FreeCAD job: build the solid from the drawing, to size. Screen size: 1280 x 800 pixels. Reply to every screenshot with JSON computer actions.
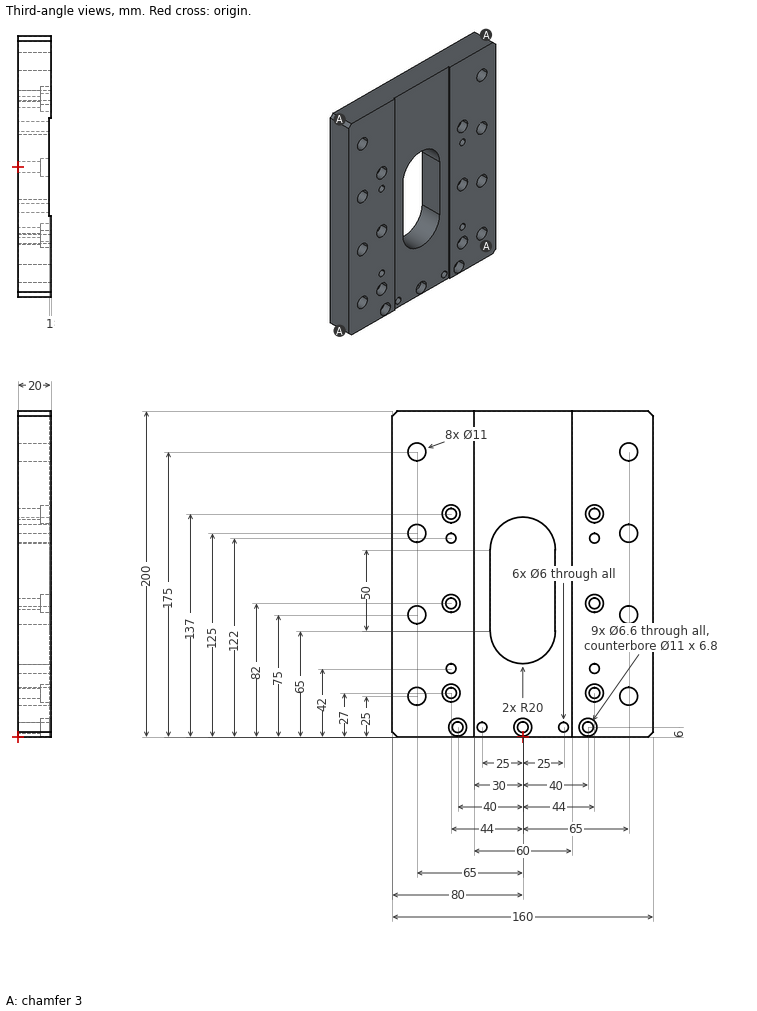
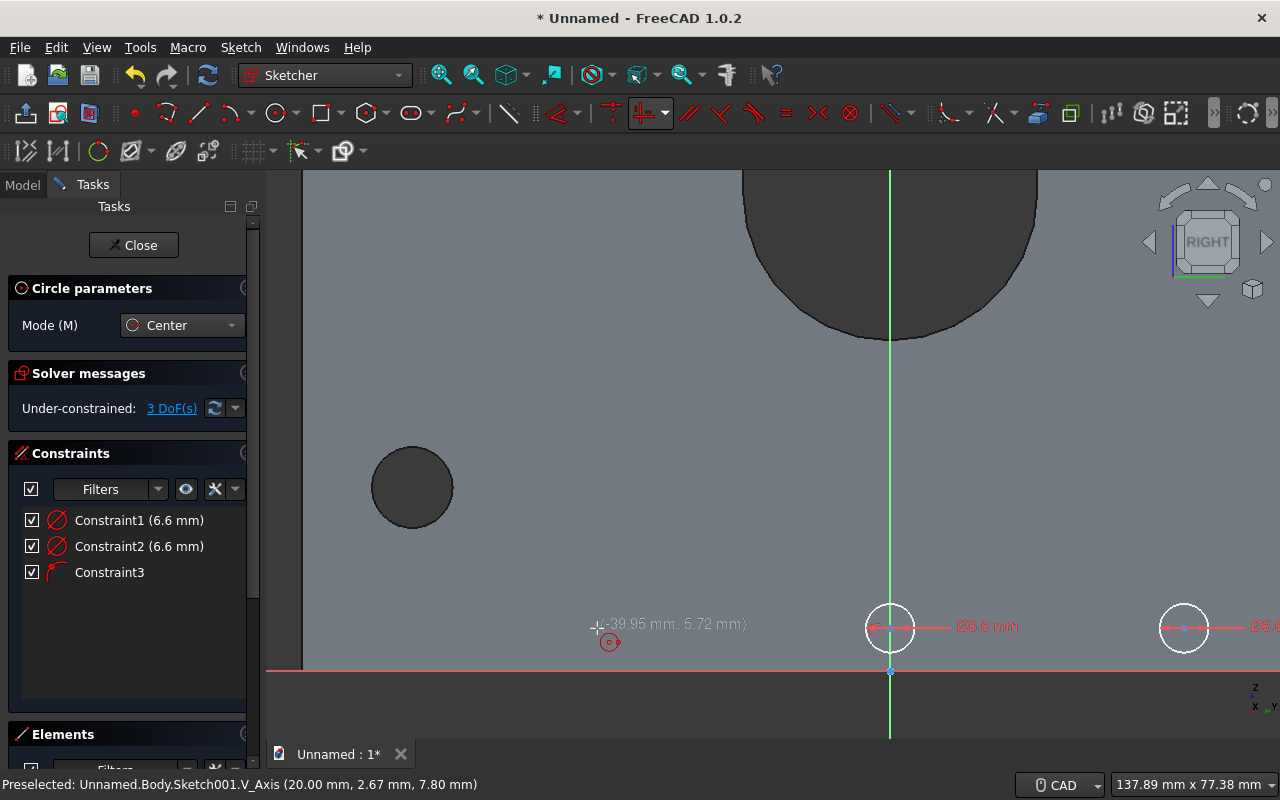
{"action": "left_click", "coordinate": [596, 627]}
{"action": "mouse_move", "coordinate": [613, 610]}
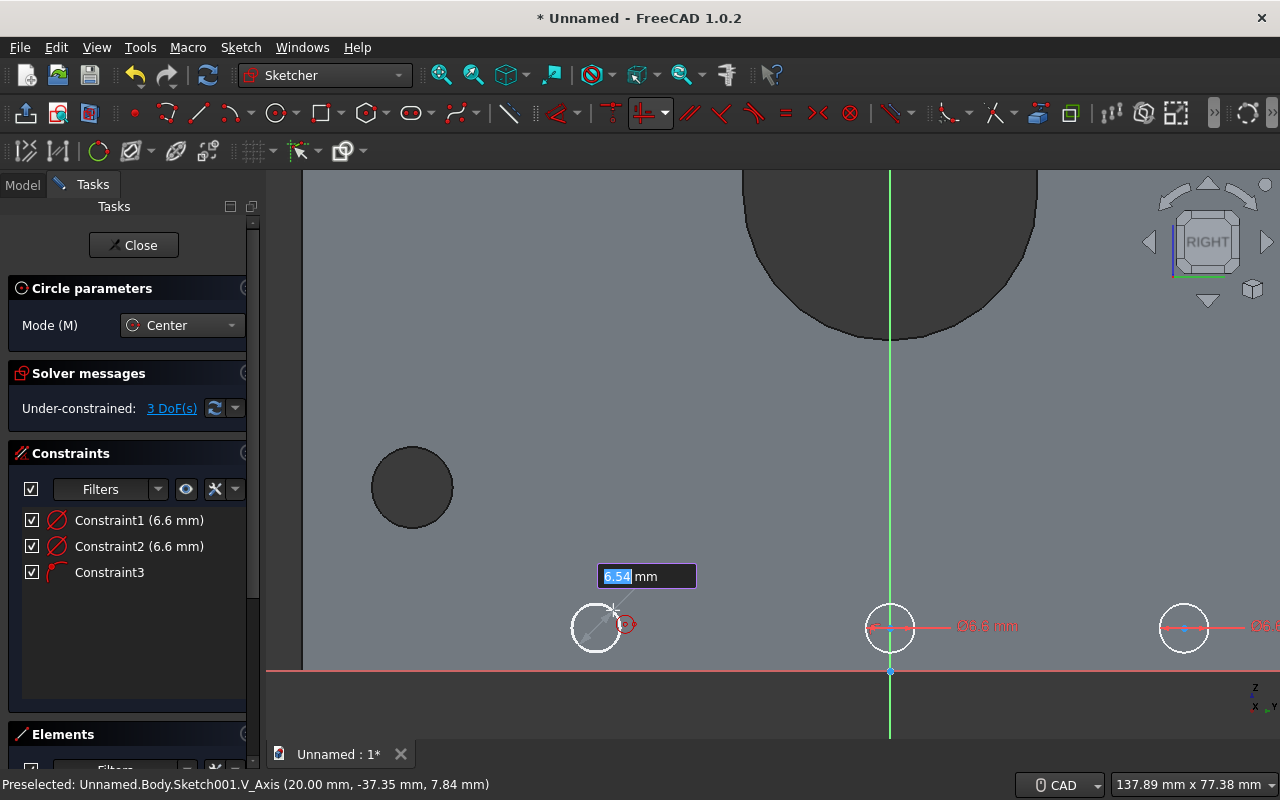
{"action": "type", "text": "6.6"}
{"action": "key", "text": "Return"}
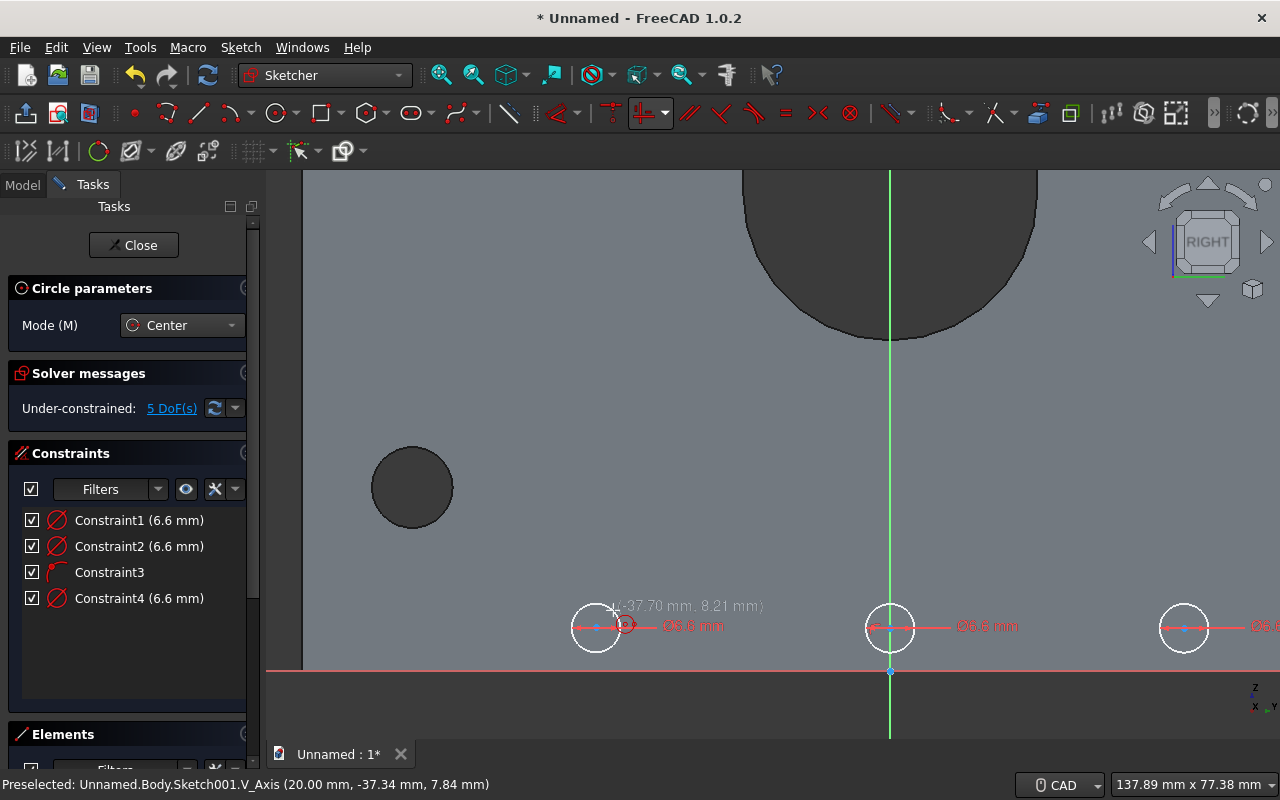
{"action": "left_click", "coordinate": [567, 473]}
{"action": "mouse_move", "coordinate": [584, 456]}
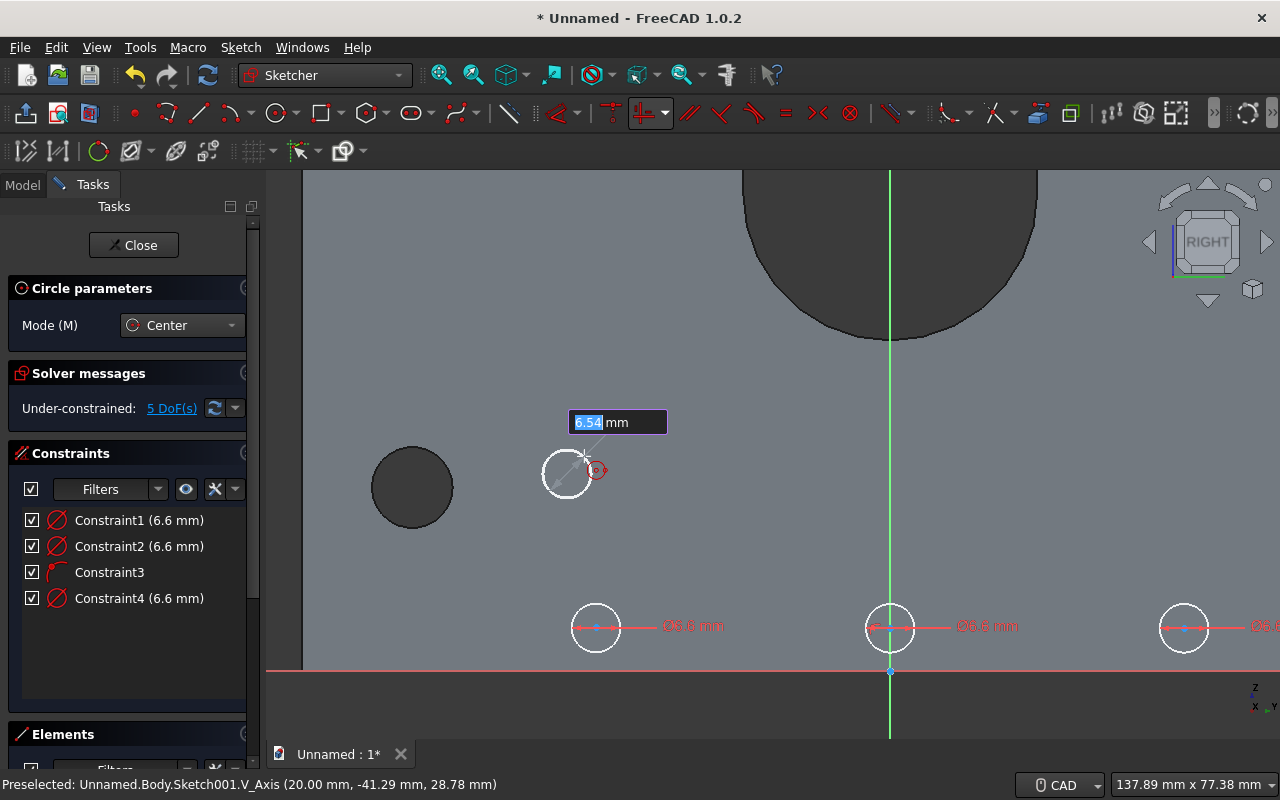
{"action": "type", "text": "6.6"}
{"action": "key", "text": "Return"}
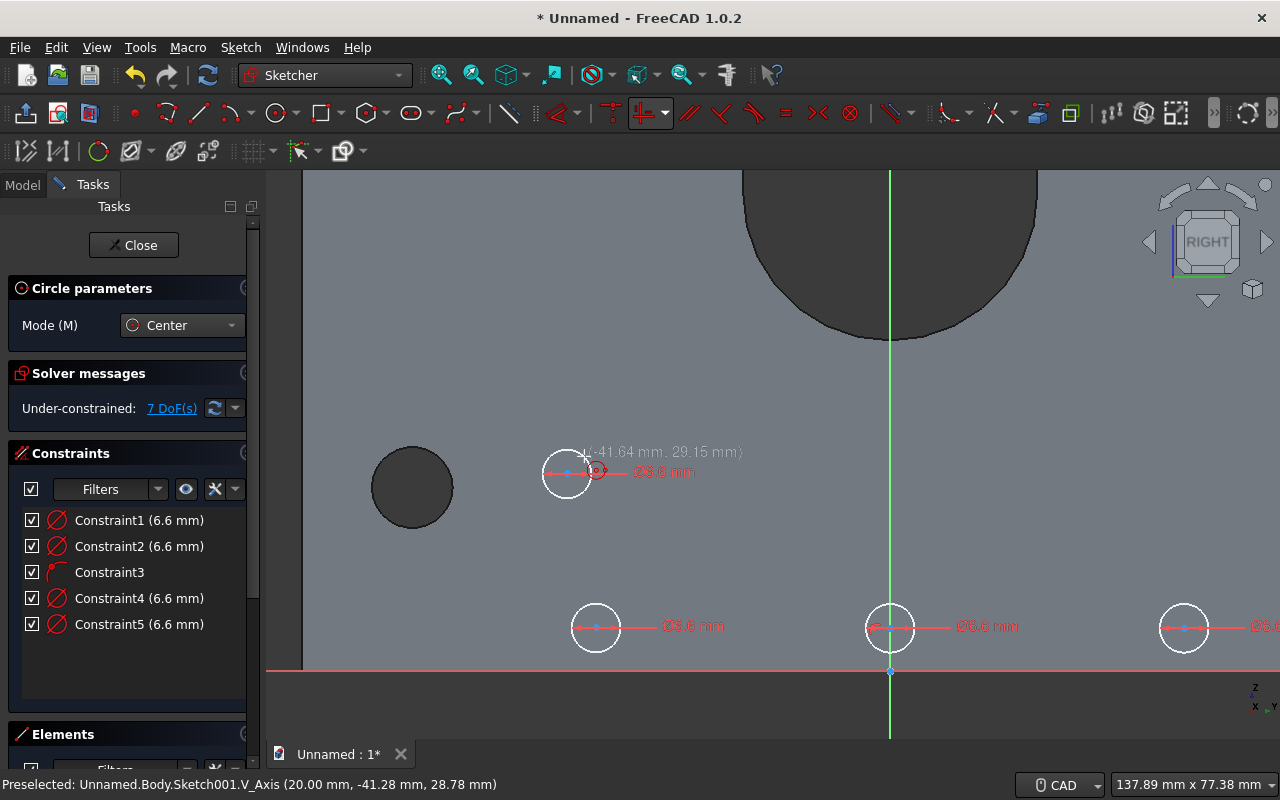
{"action": "scroll", "coordinate": [596, 628], "scroll_direction": "down", "scroll_amount": 5}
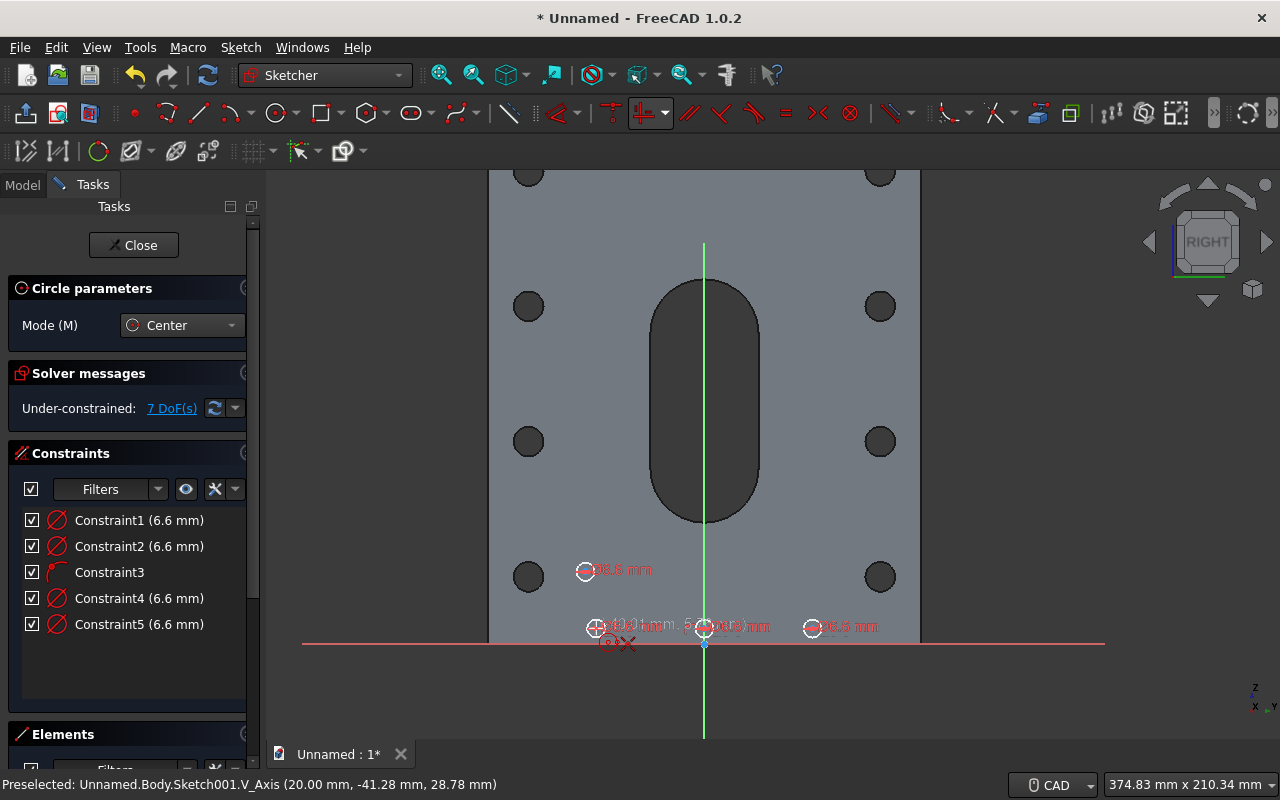
{"action": "scroll", "coordinate": [585, 423], "scroll_direction": "up", "scroll_amount": 5}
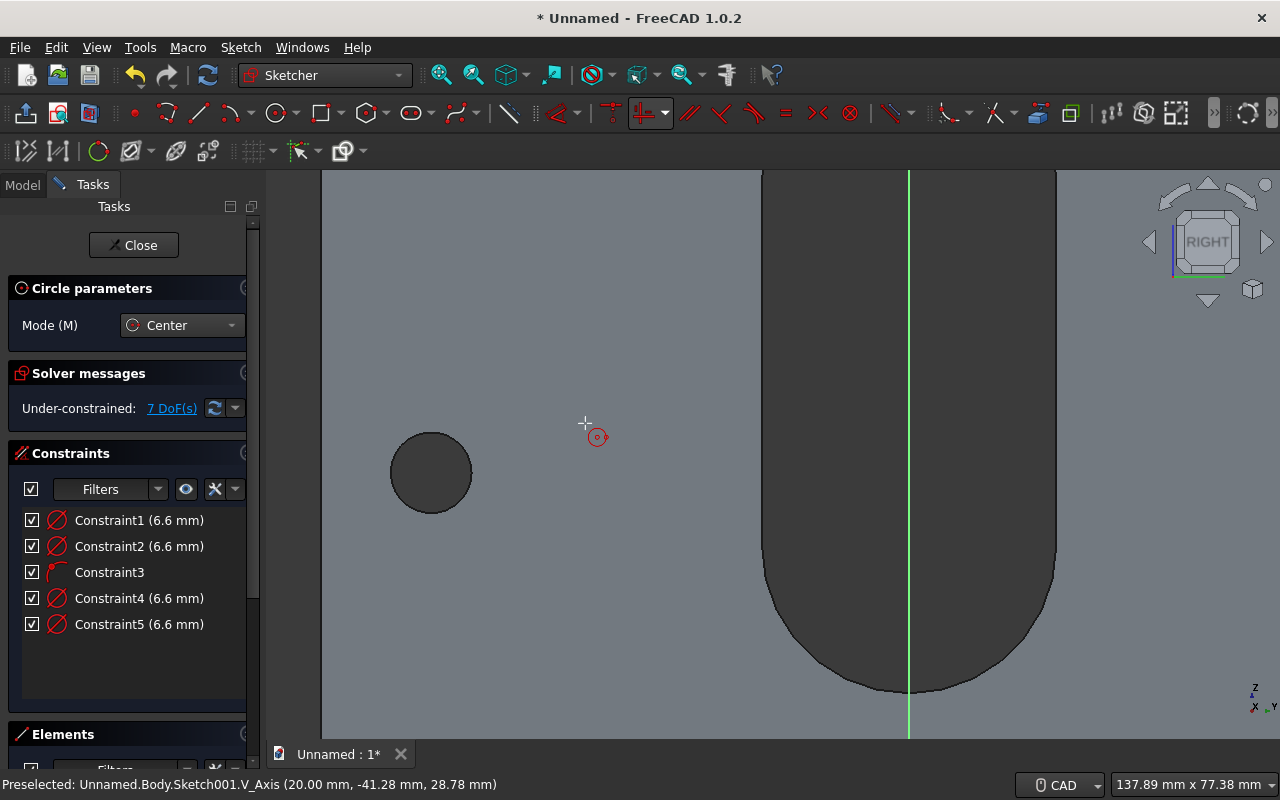
{"action": "left_click", "coordinate": [586, 421]}
{"action": "mouse_move", "coordinate": [603, 404]}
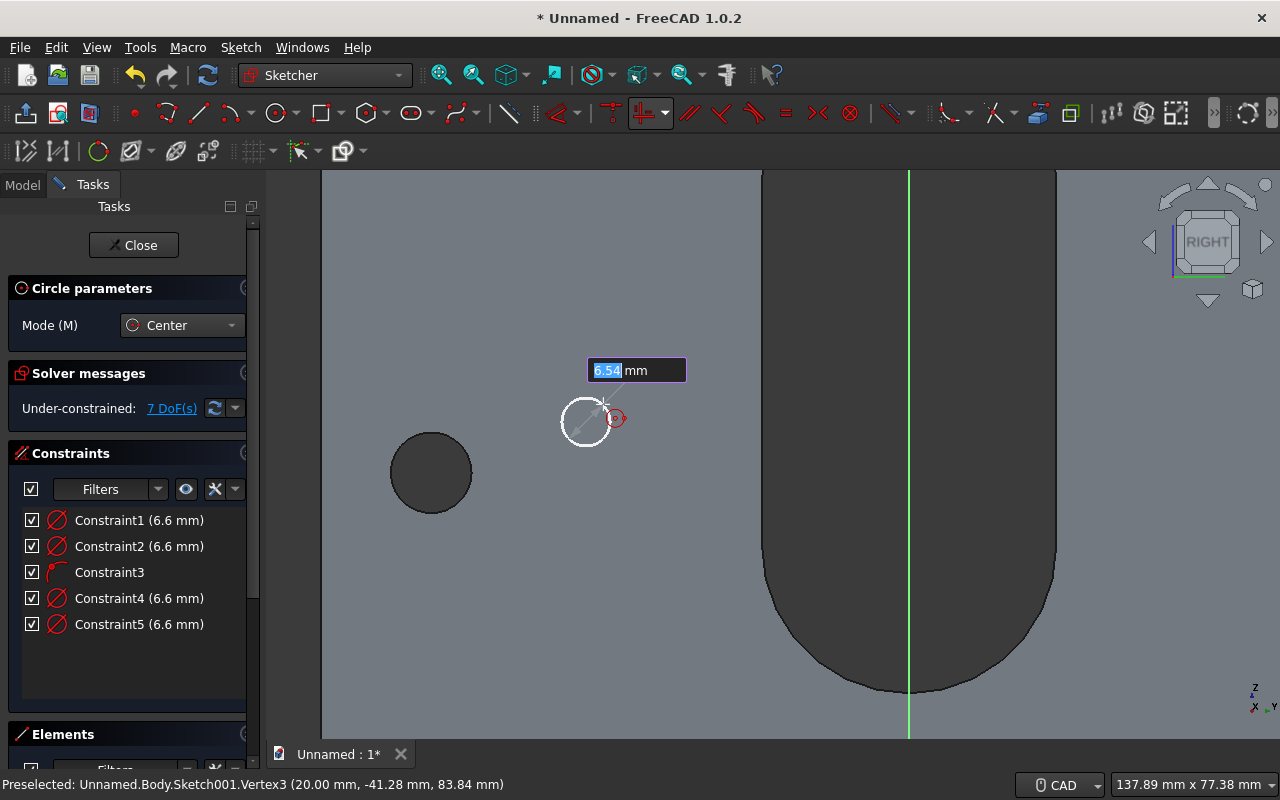
{"action": "type", "text": "6.6"}
{"action": "key", "text": "Return"}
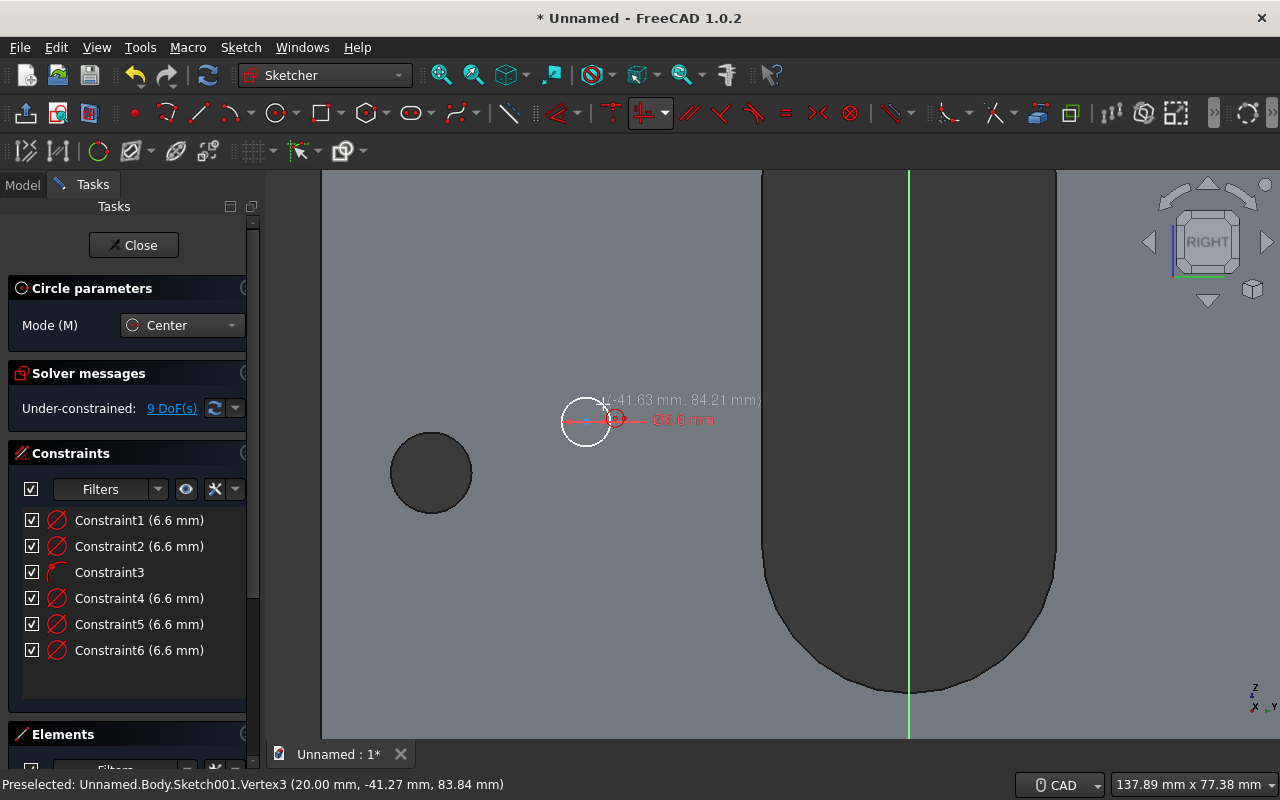
{"action": "scroll", "coordinate": [585, 423], "scroll_direction": "down", "scroll_amount": 5}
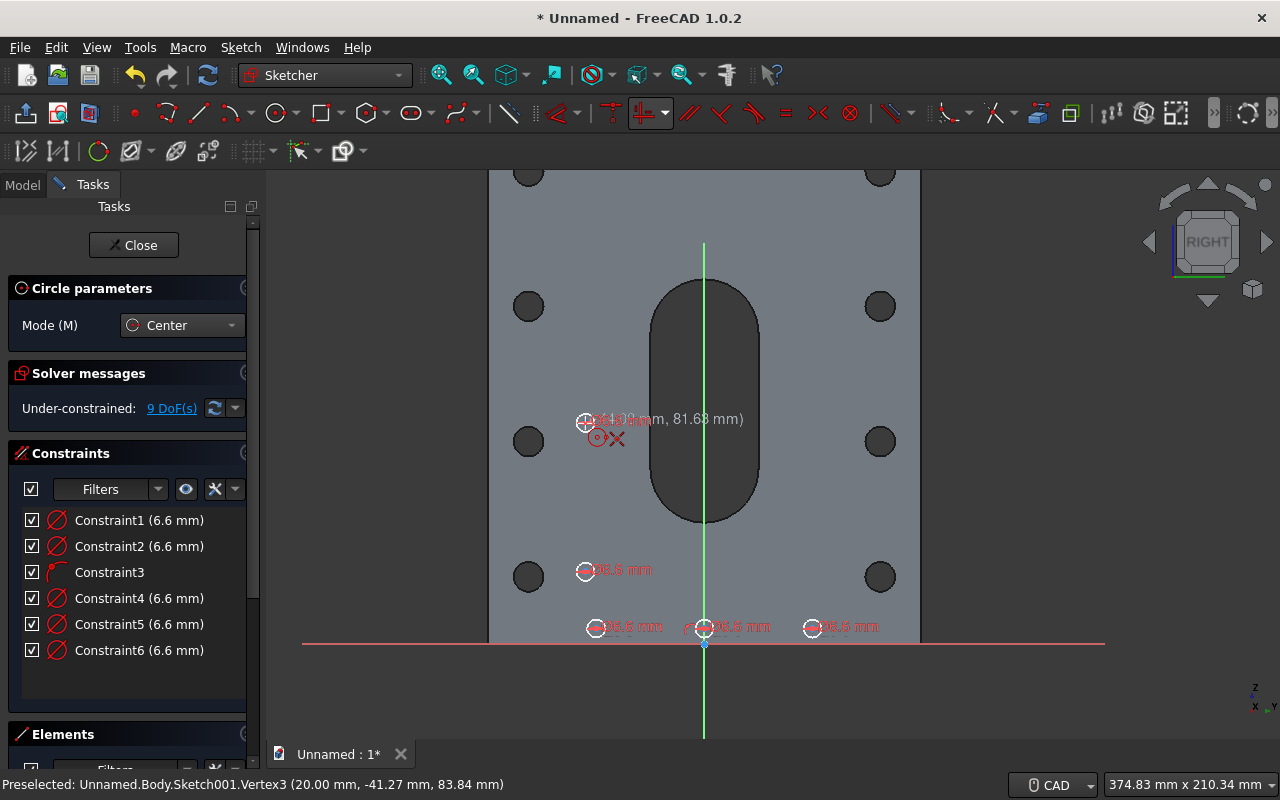
{"action": "scroll", "coordinate": [585, 274], "scroll_direction": "up", "scroll_amount": 5}